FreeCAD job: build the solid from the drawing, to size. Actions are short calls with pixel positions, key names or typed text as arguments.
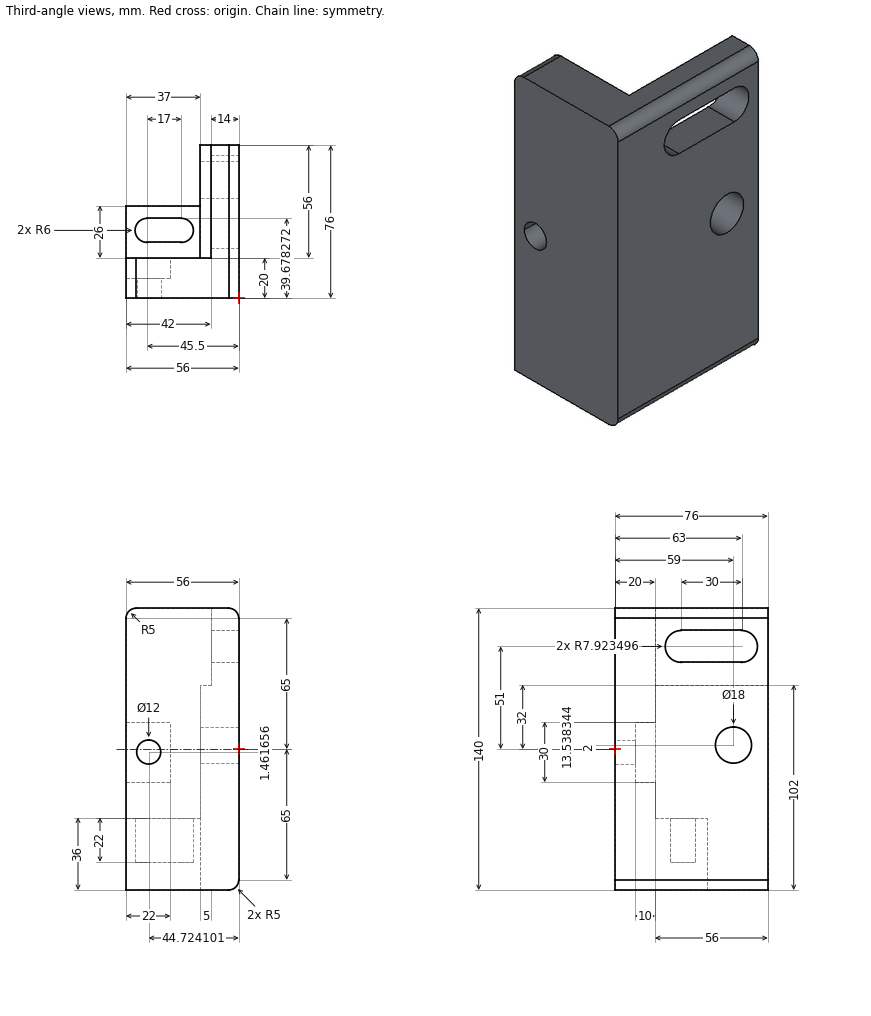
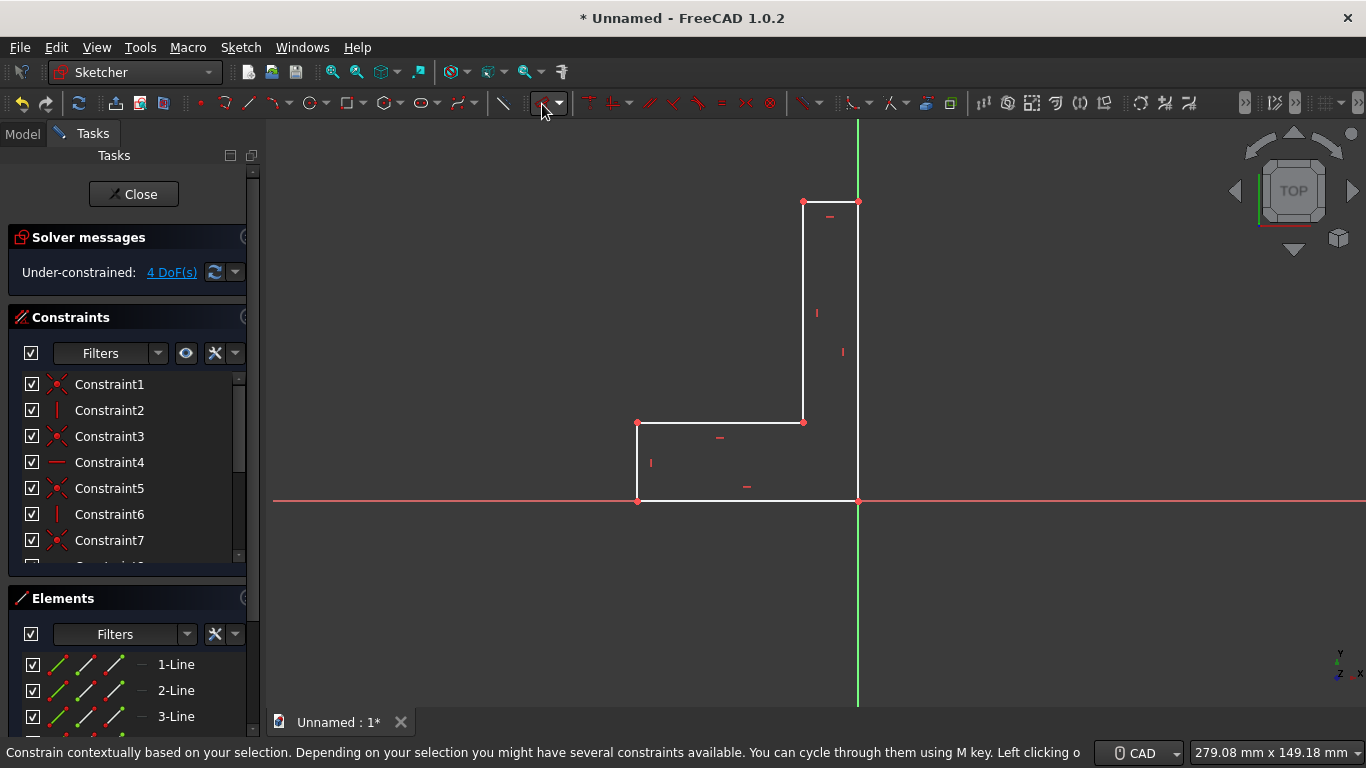
click(858, 411)
click(892, 352)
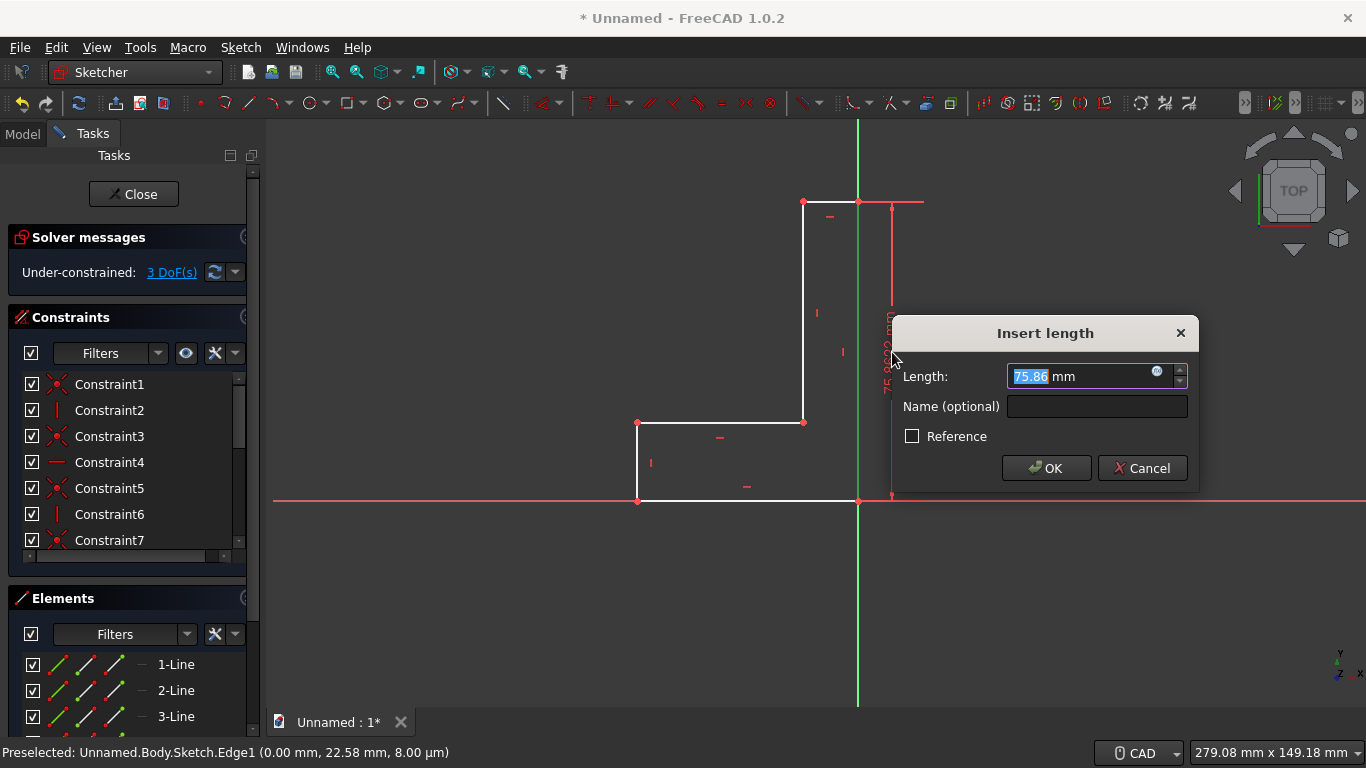
text(76)
key(Return)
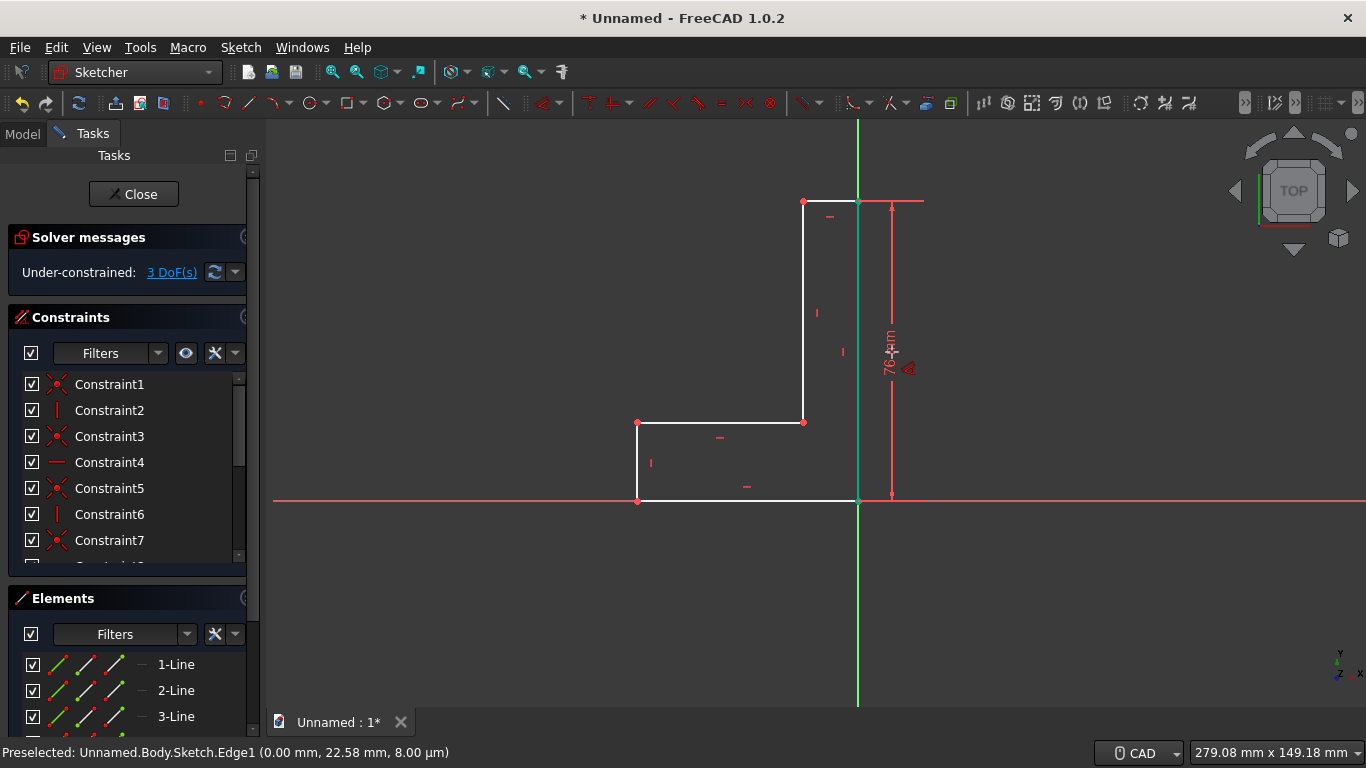
click(842, 201)
click(831, 167)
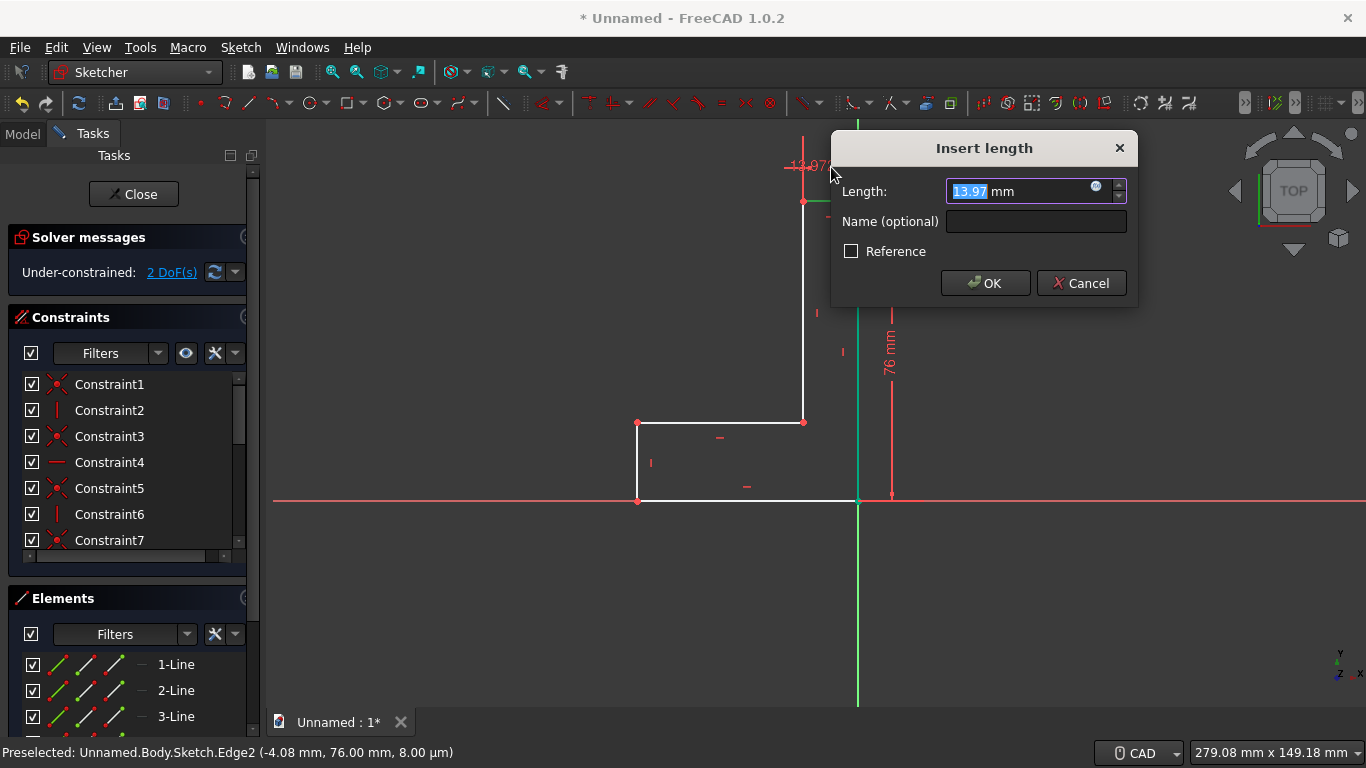
text(14)
key(Return)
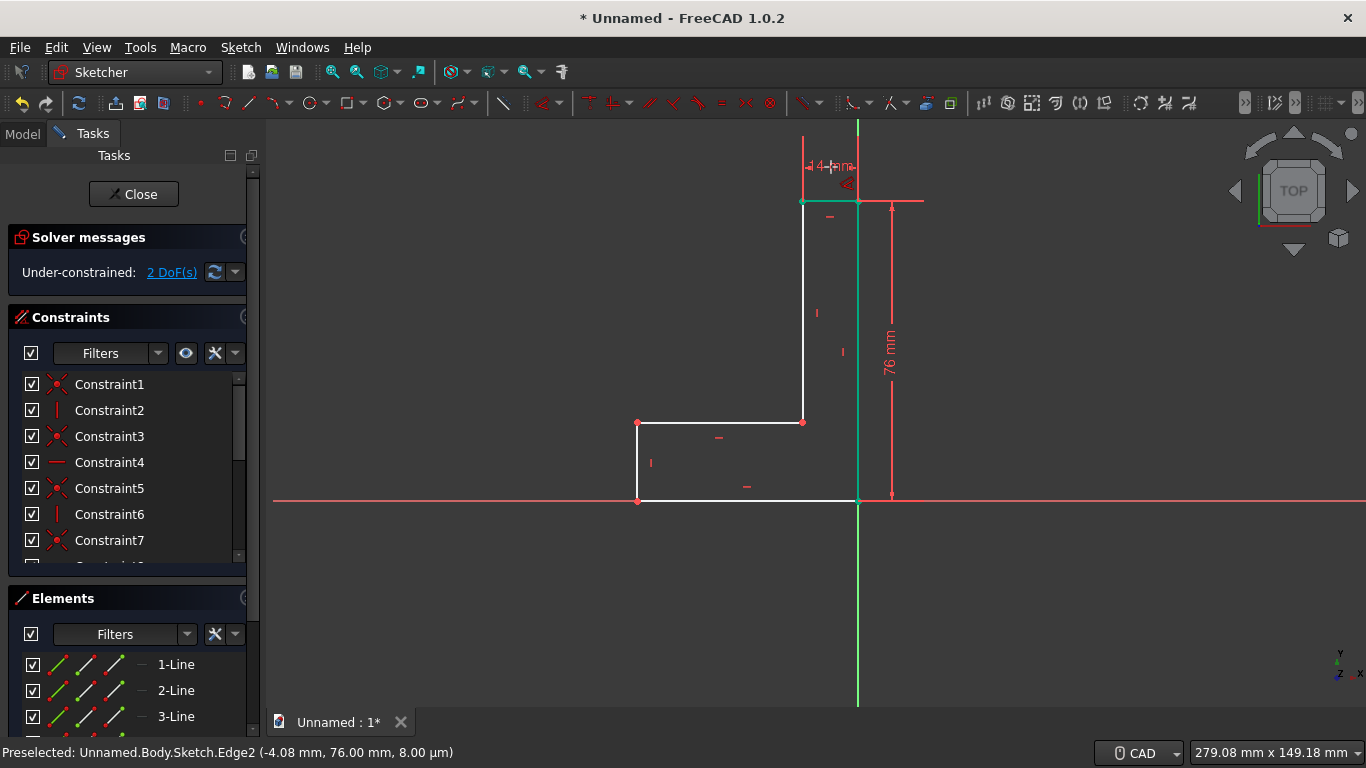
click(803, 268)
click(837, 312)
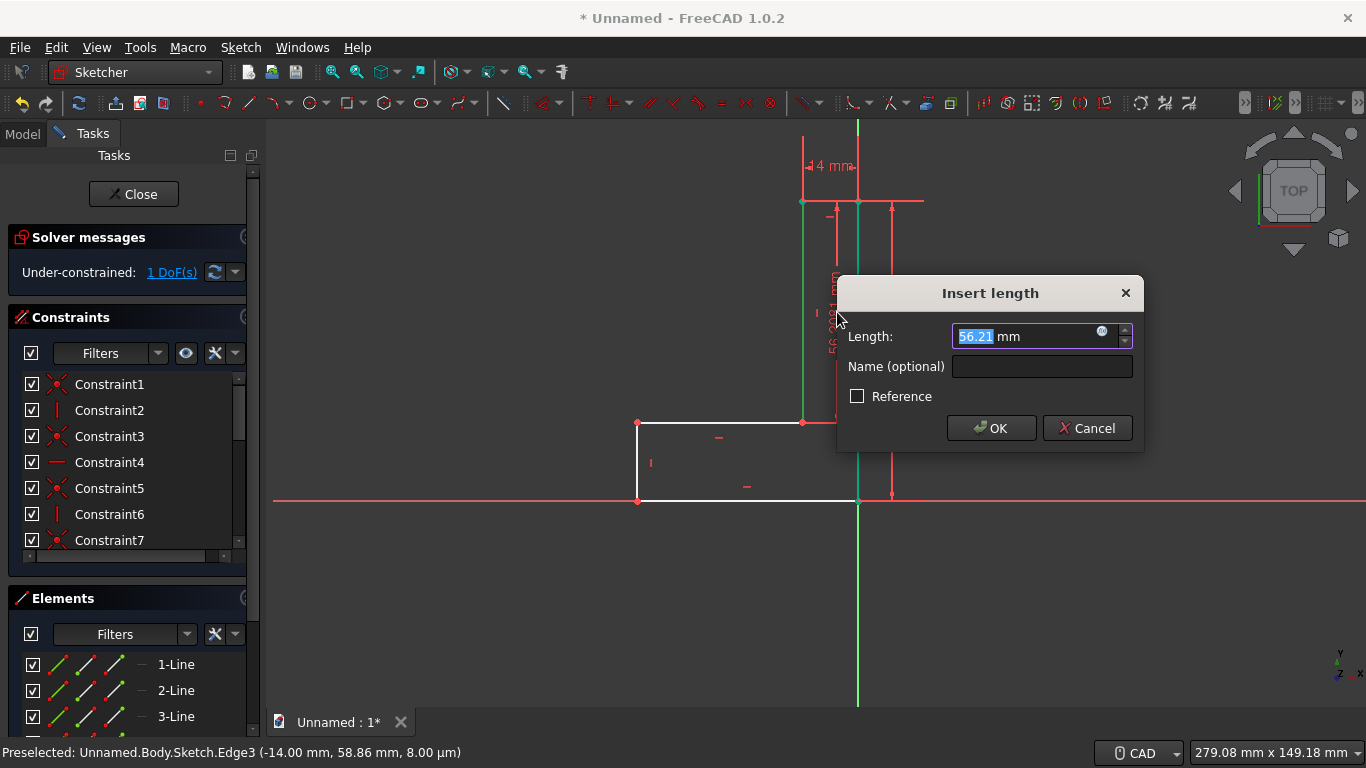
text(56)
key(Return)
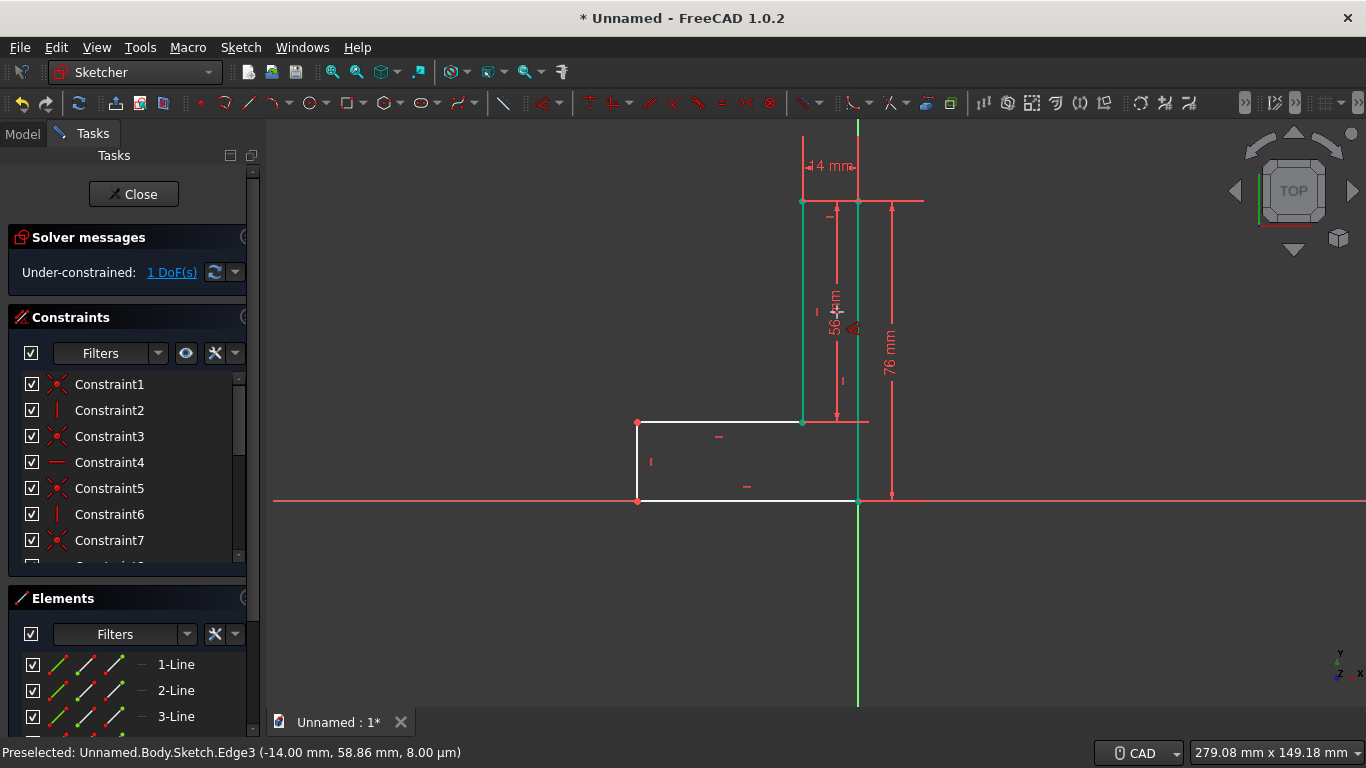
click(753, 422)
click(720, 456)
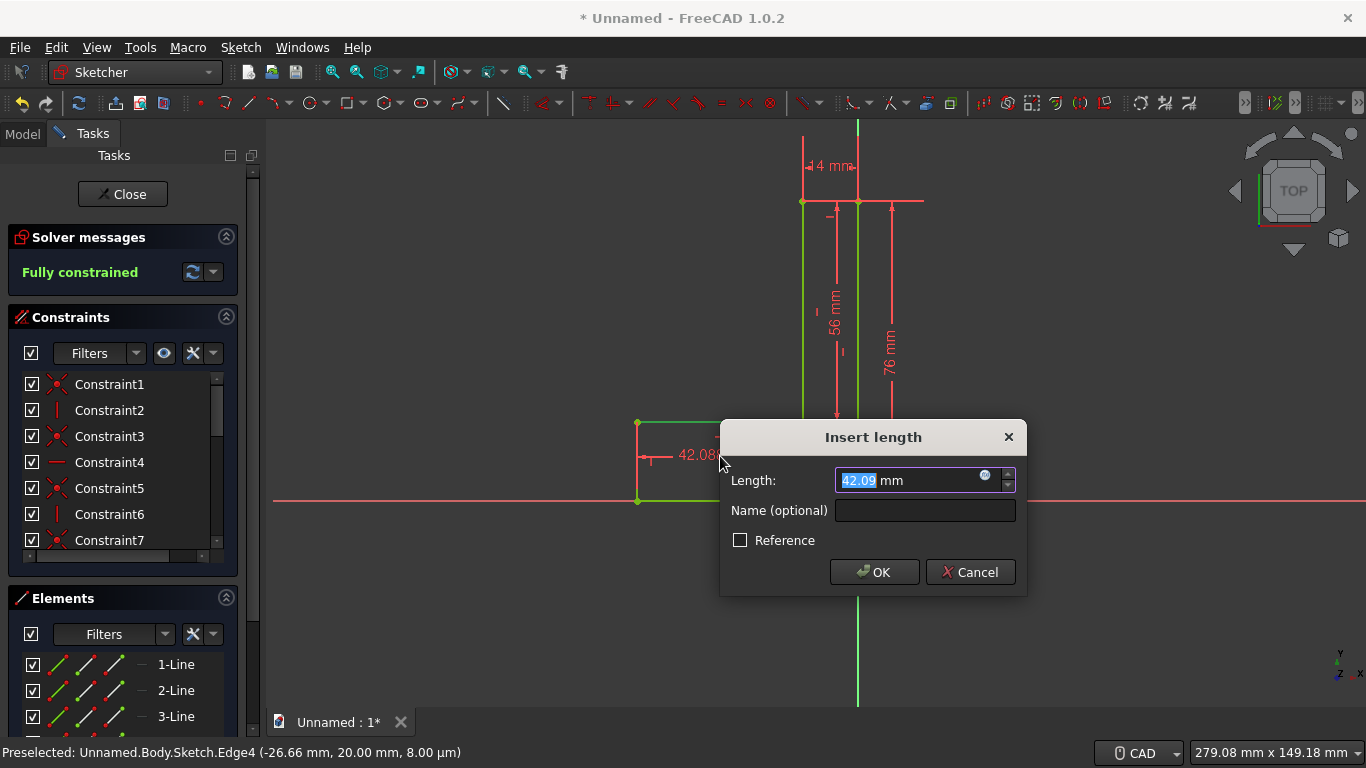
text(42)
key(Return)
key(Escape)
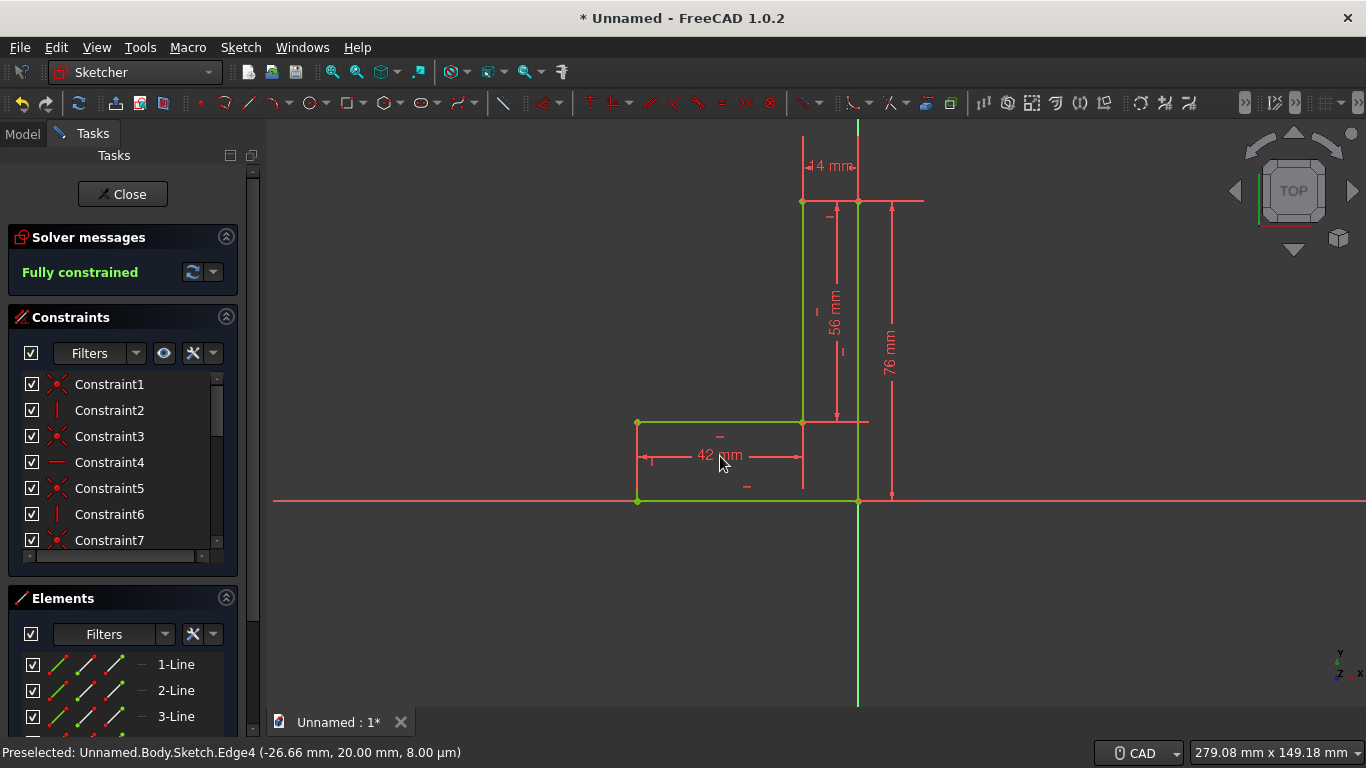
click(123, 194)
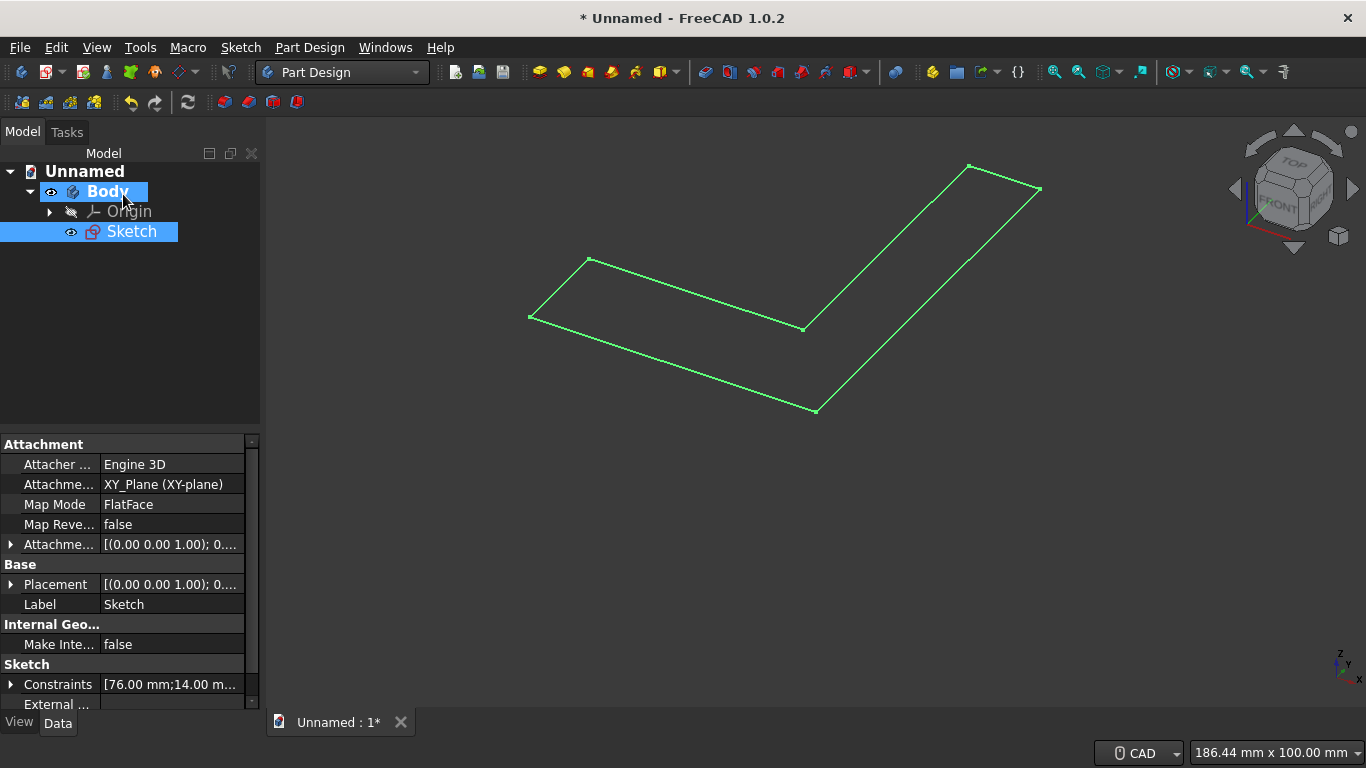
click(540, 72)